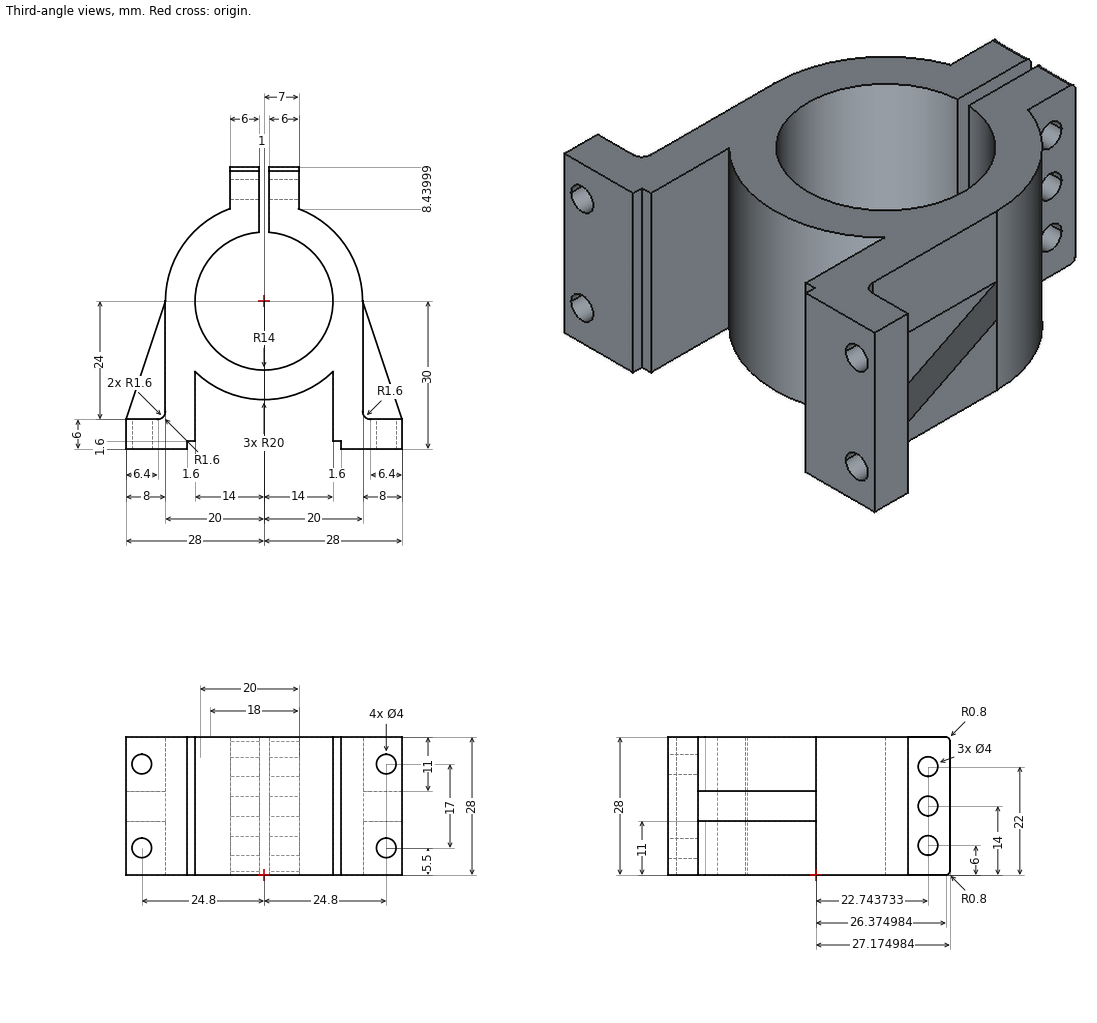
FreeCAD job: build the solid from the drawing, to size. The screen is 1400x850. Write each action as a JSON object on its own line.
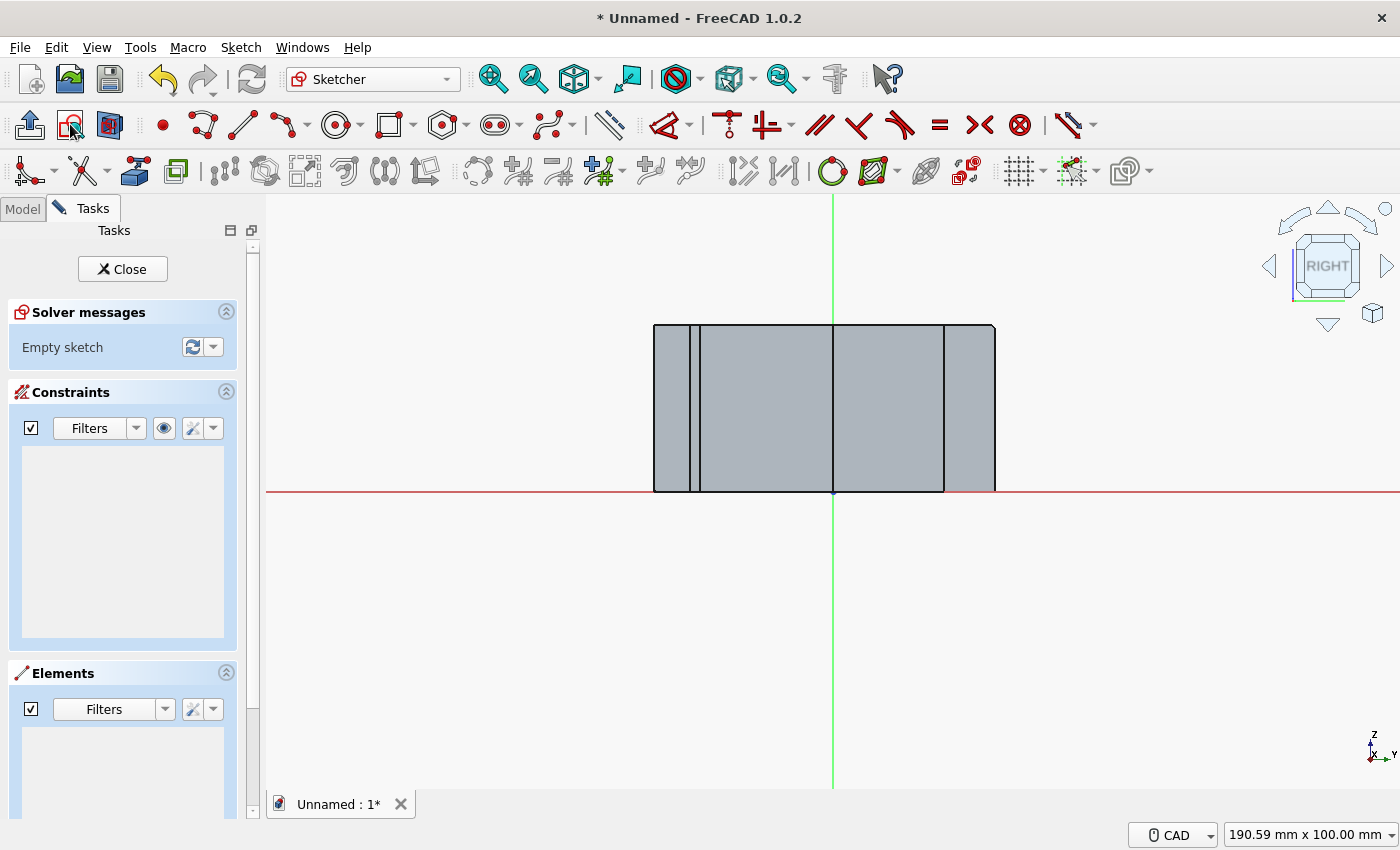
{"action": "scroll", "coordinate": [1004, 489], "scroll_direction": "up", "scroll_amount": 15}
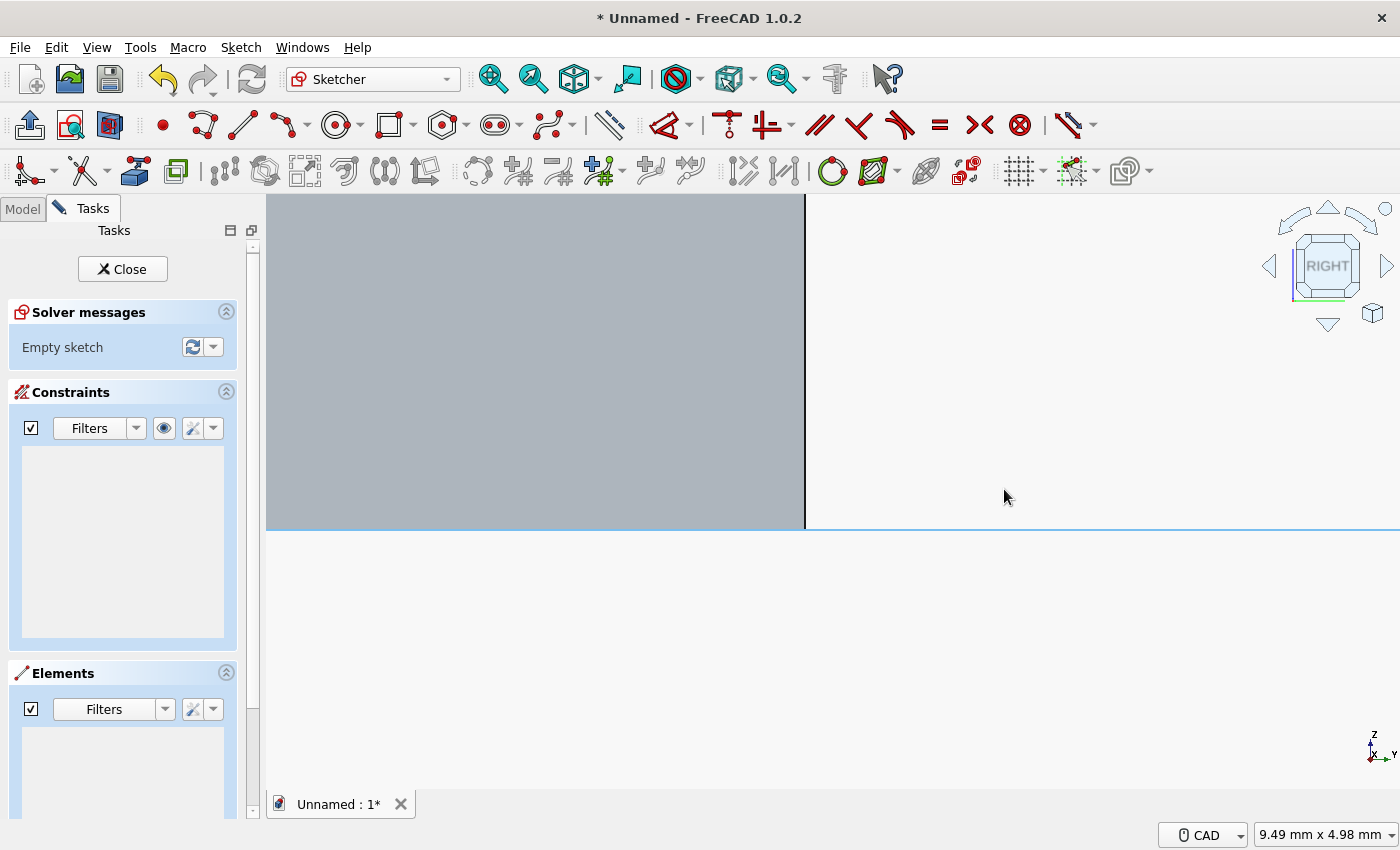
{"action": "scroll", "coordinate": [754, 479], "scroll_direction": "up", "scroll_amount": 7}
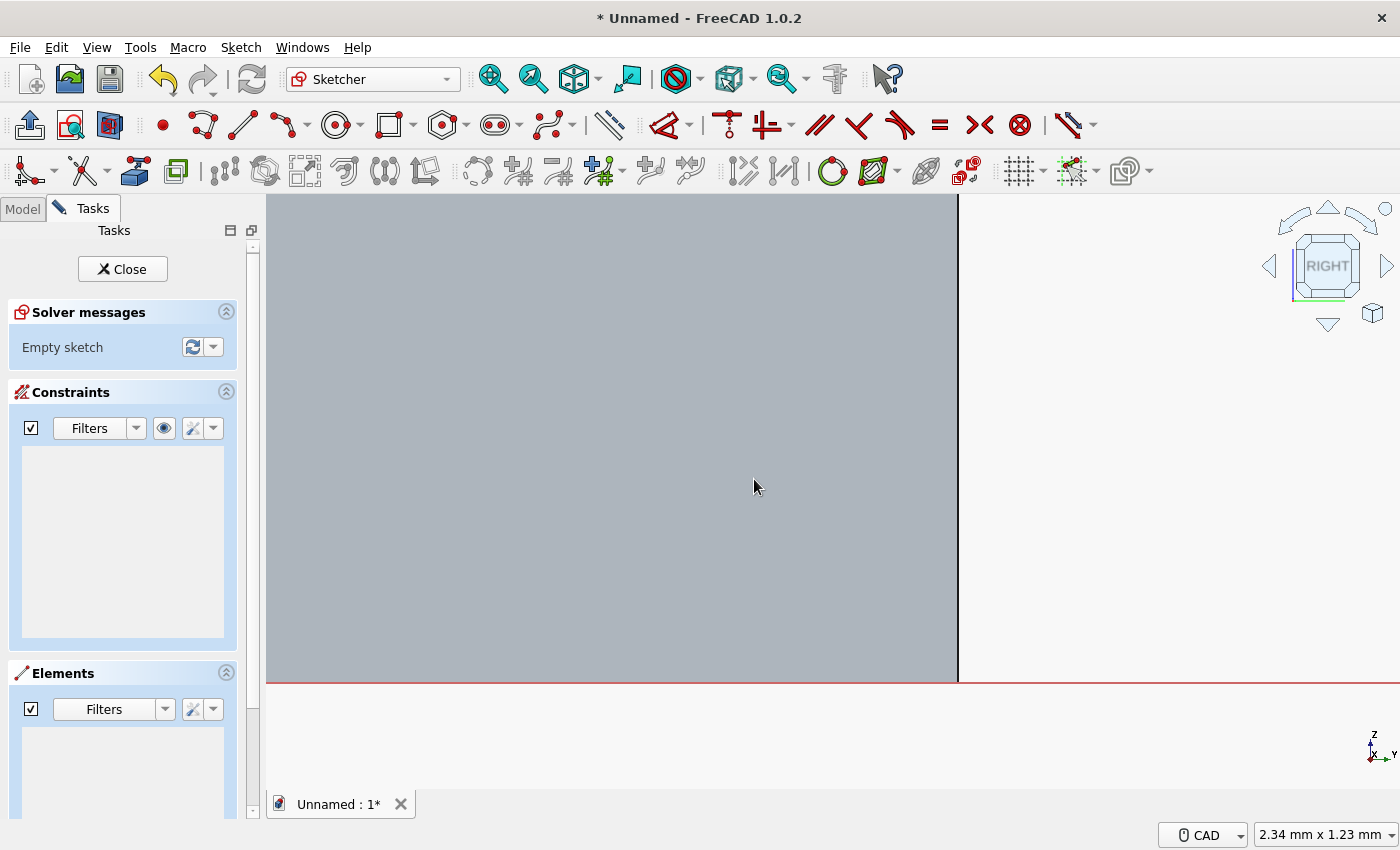
{"action": "left_click", "coordinate": [204, 126]}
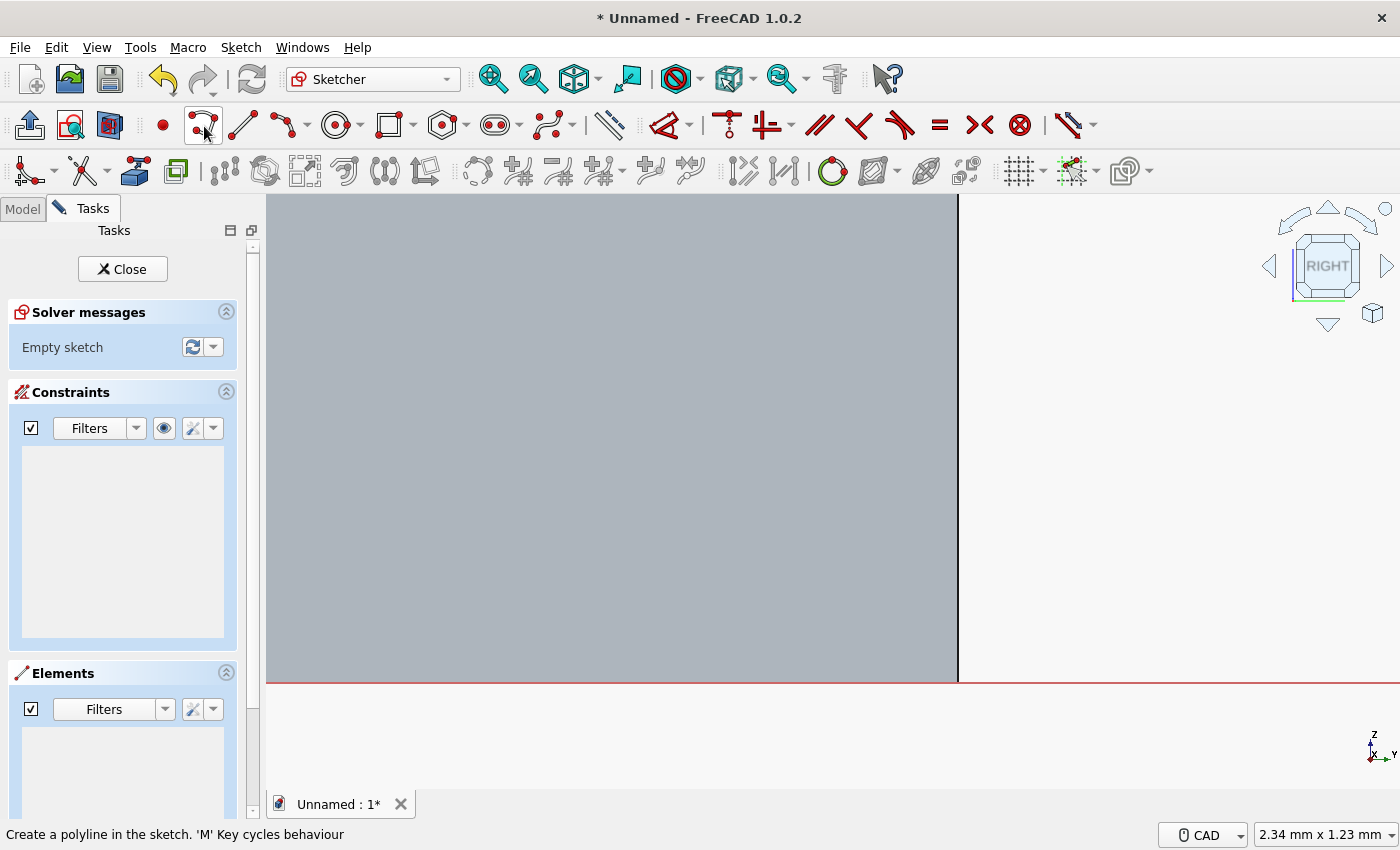
{"action": "left_click", "coordinate": [570, 683]}
{"action": "left_click", "coordinate": [958, 674]}
{"action": "left_click", "coordinate": [958, 296]}
{"action": "right_click", "coordinate": [958, 296]}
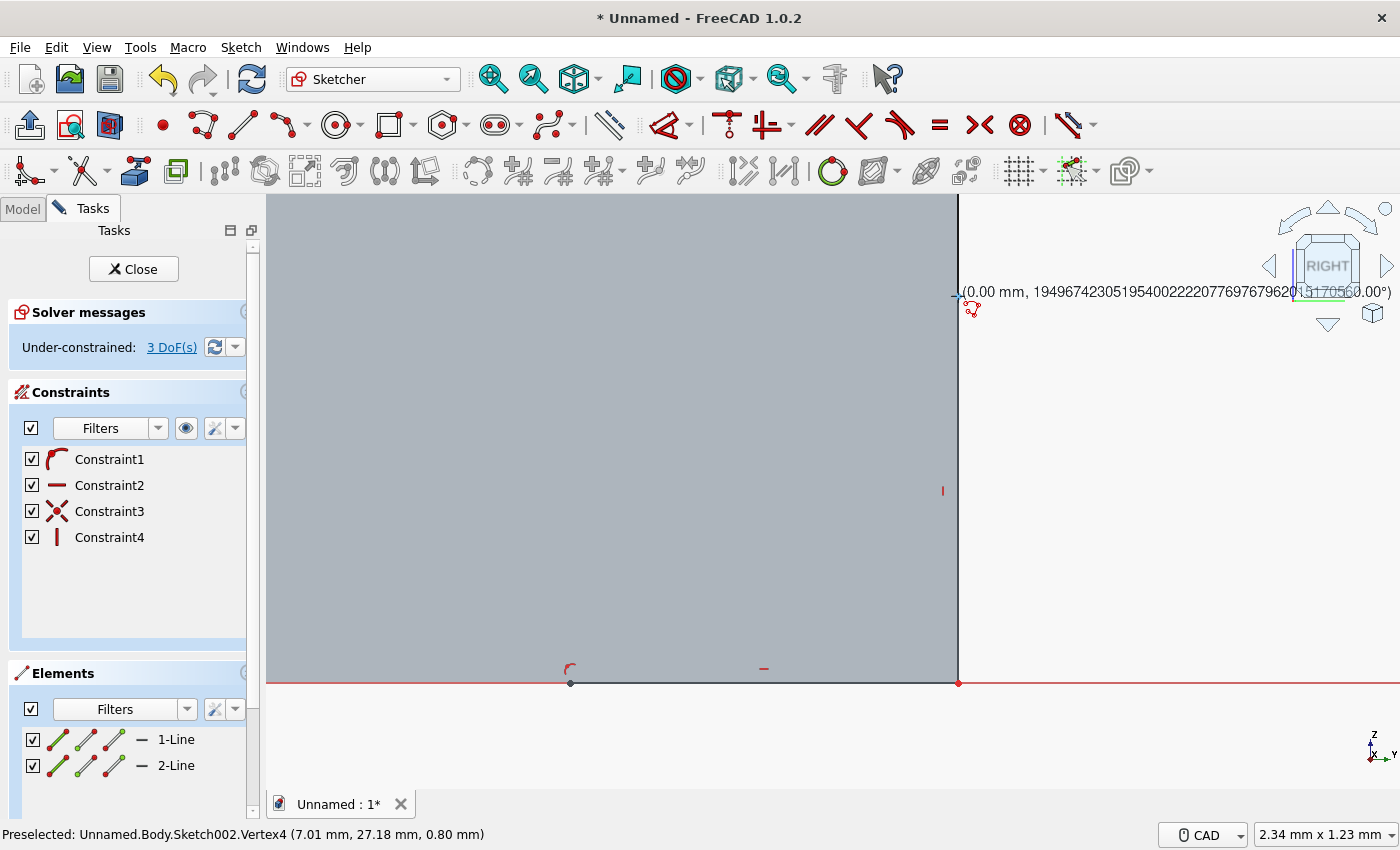
{"action": "left_click", "coordinate": [284, 126]}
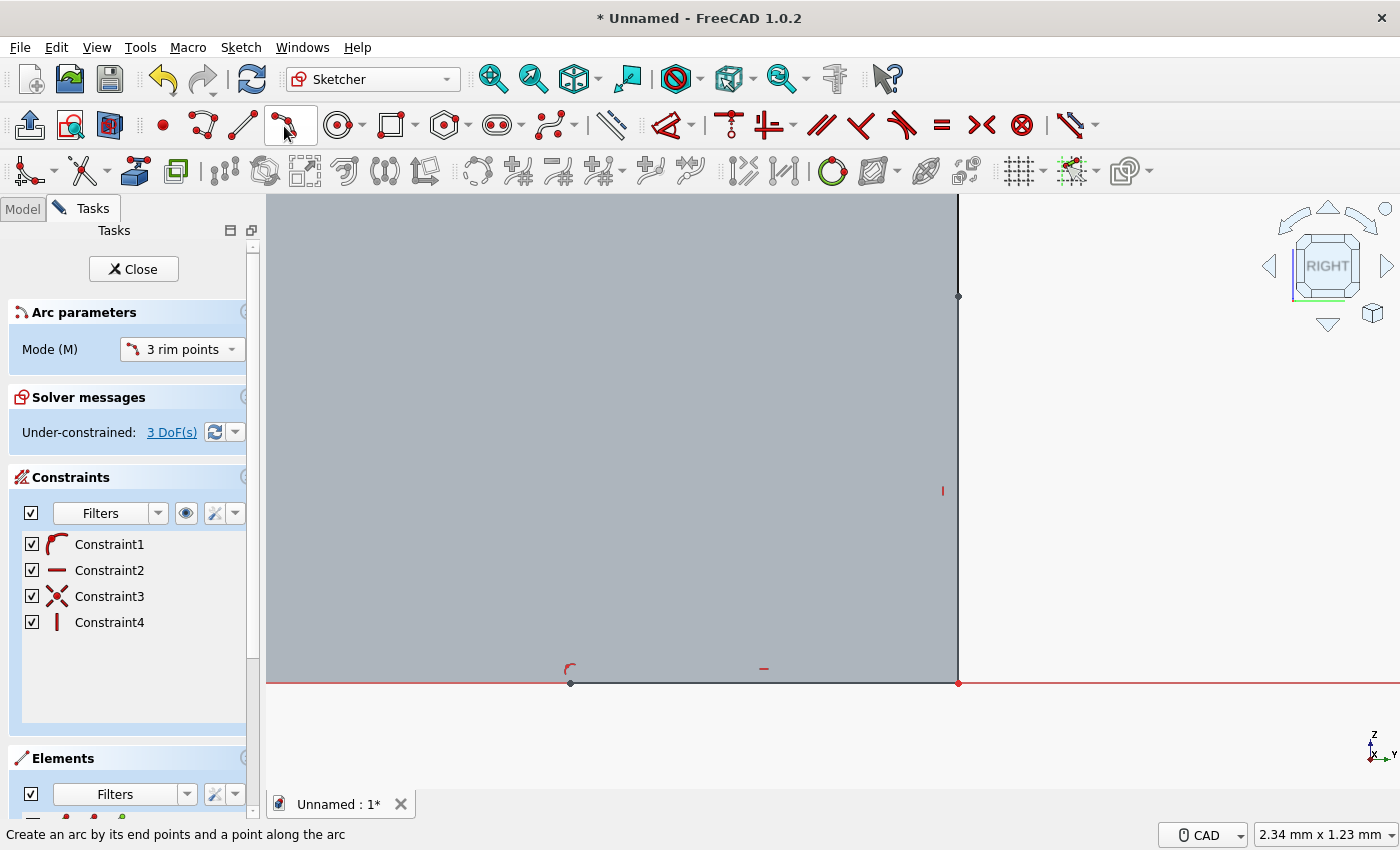
{"action": "left_click", "coordinate": [958, 297]}
{"action": "left_click", "coordinate": [570, 683]}
{"action": "left_click", "coordinate": [844, 570]}
{"action": "key", "text": "Escape"}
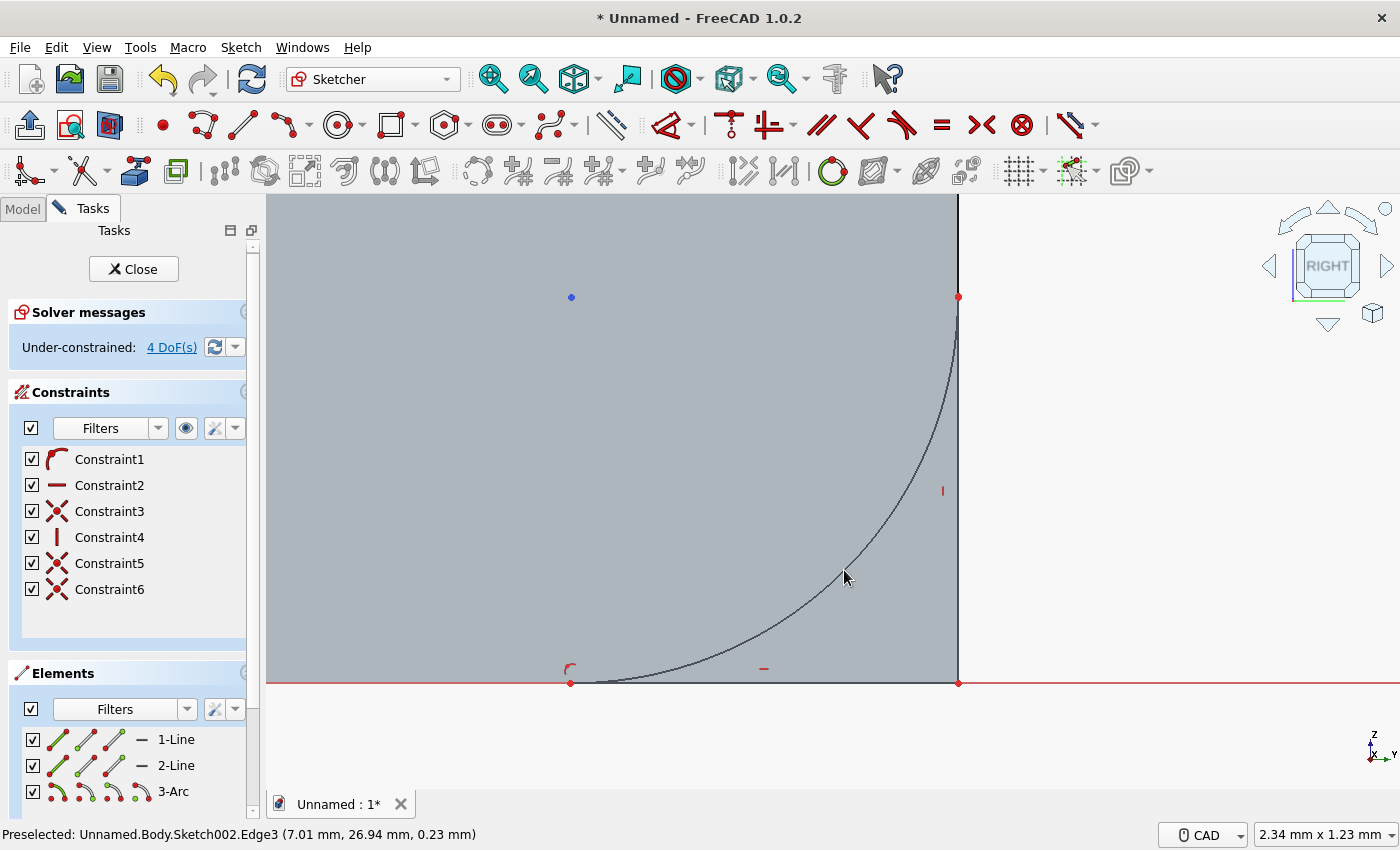
{"action": "left_click", "coordinate": [686, 683]}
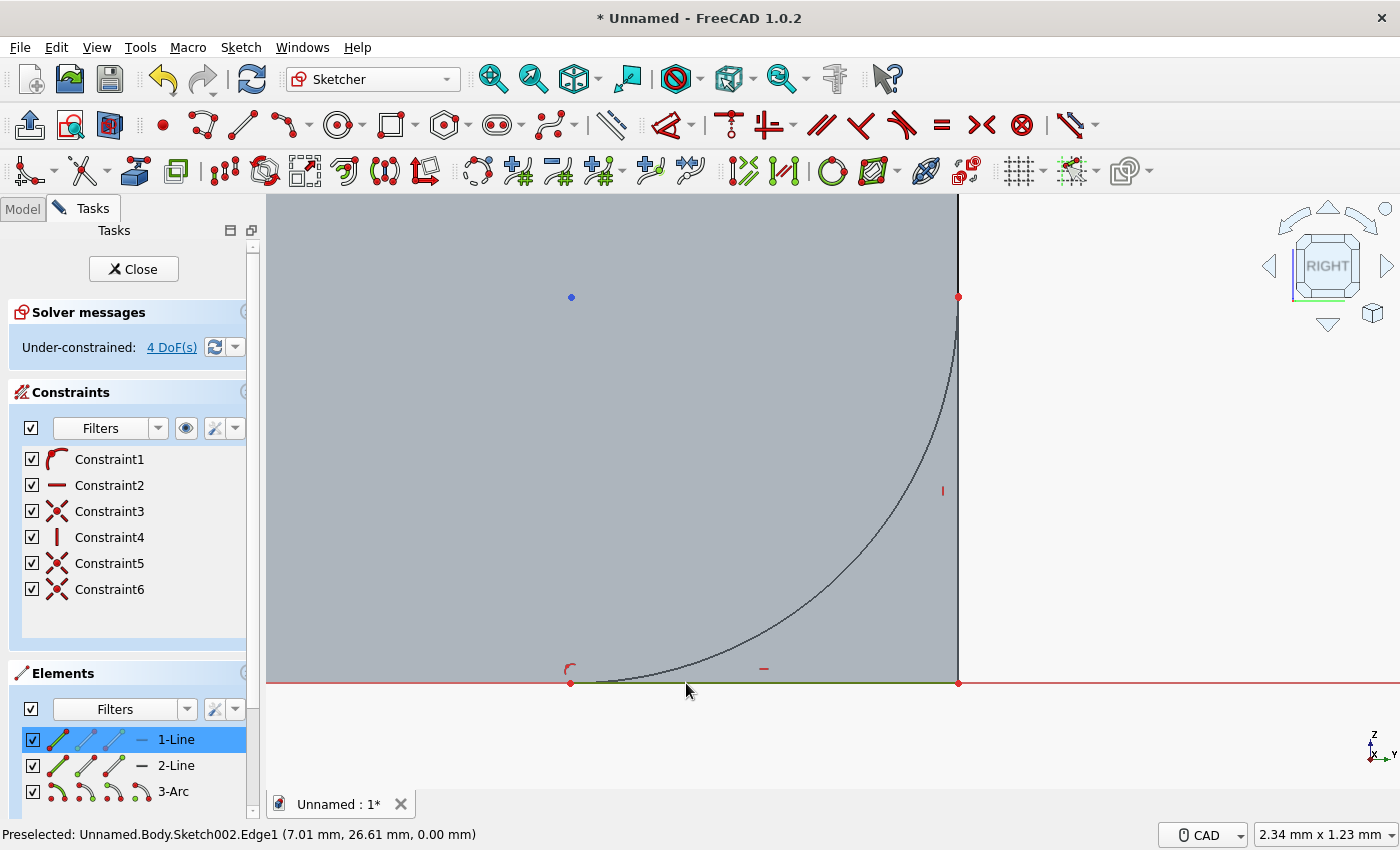
{"action": "left_click", "coordinate": [746, 642]}